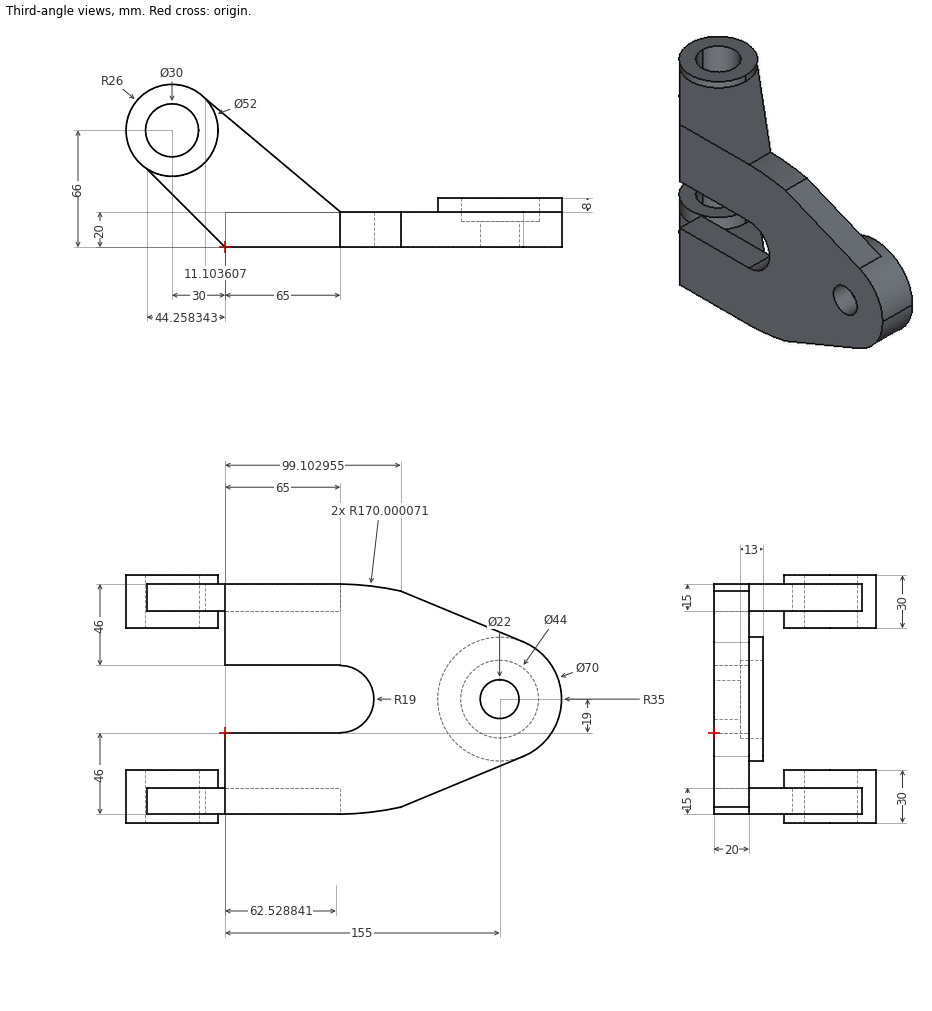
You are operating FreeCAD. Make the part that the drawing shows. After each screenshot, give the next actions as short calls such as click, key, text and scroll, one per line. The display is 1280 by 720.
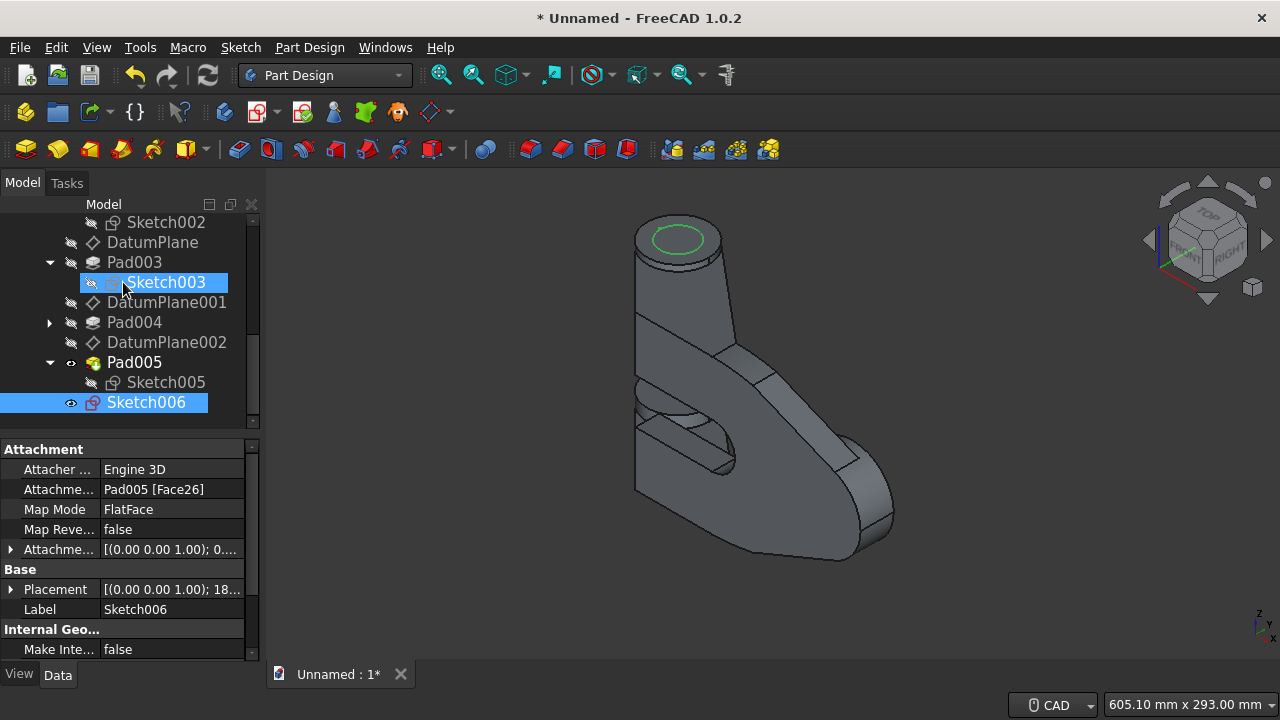
click(240, 150)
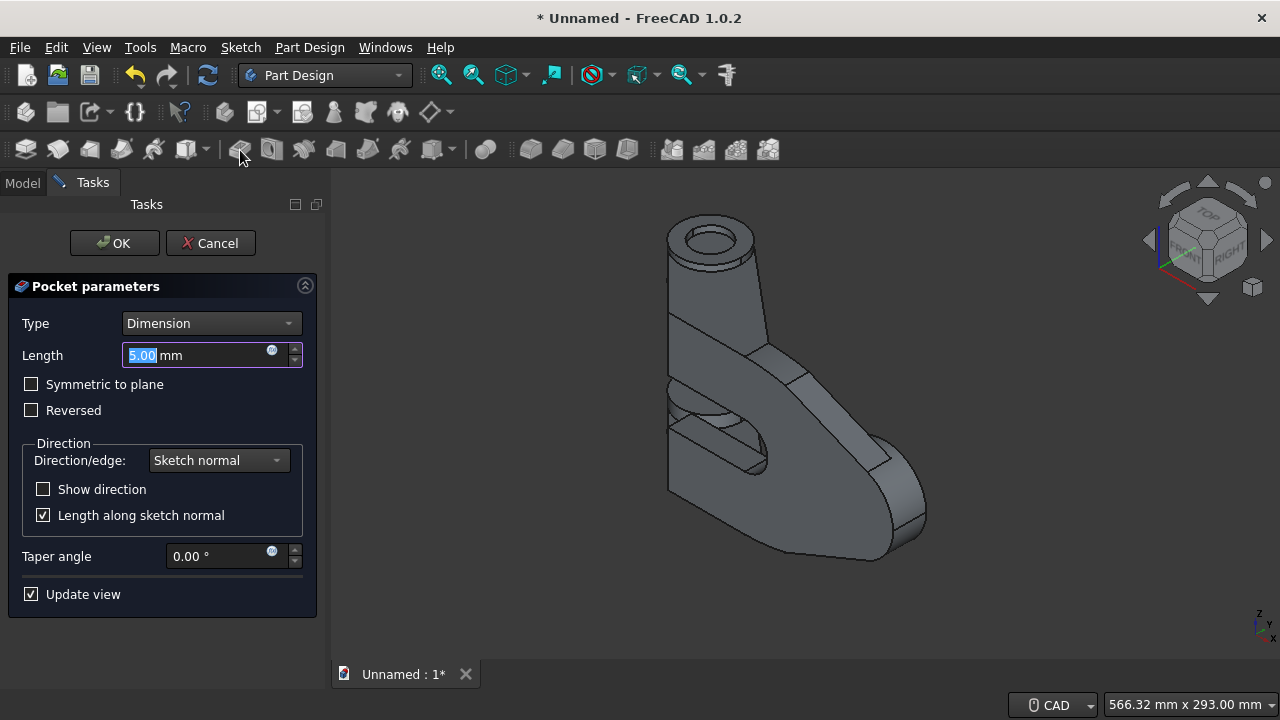
click(212, 324)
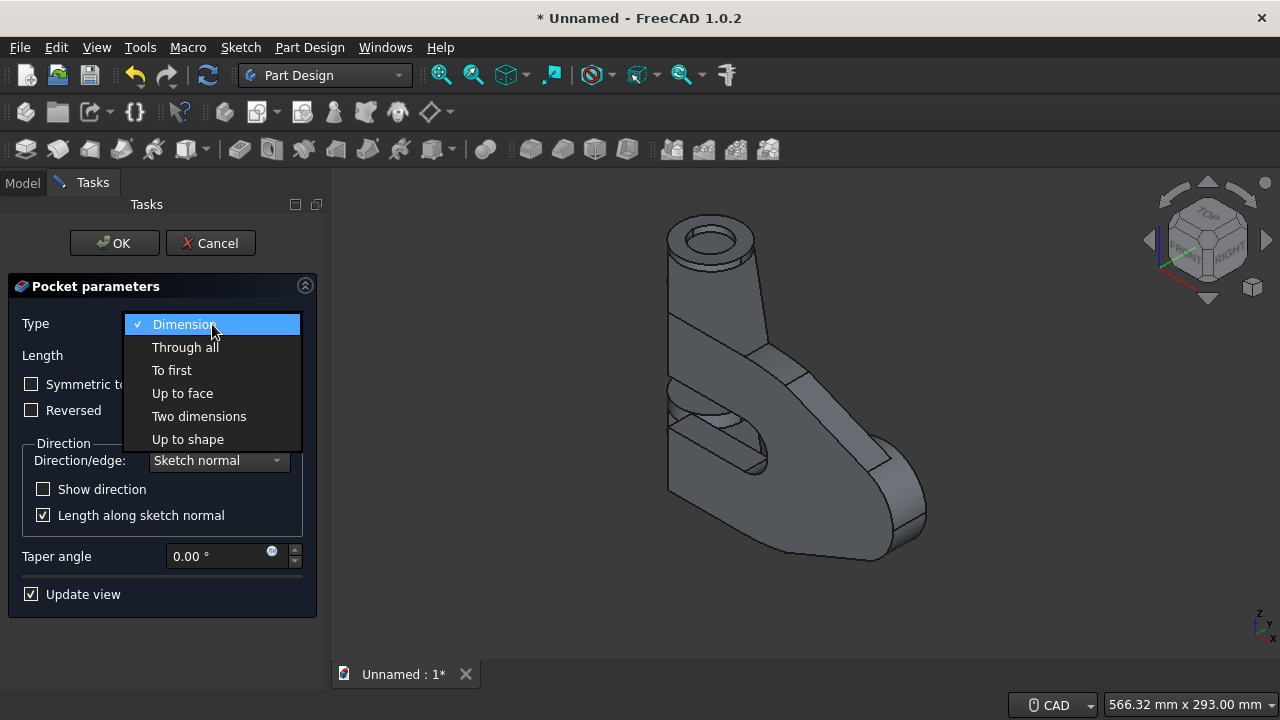
click(212, 348)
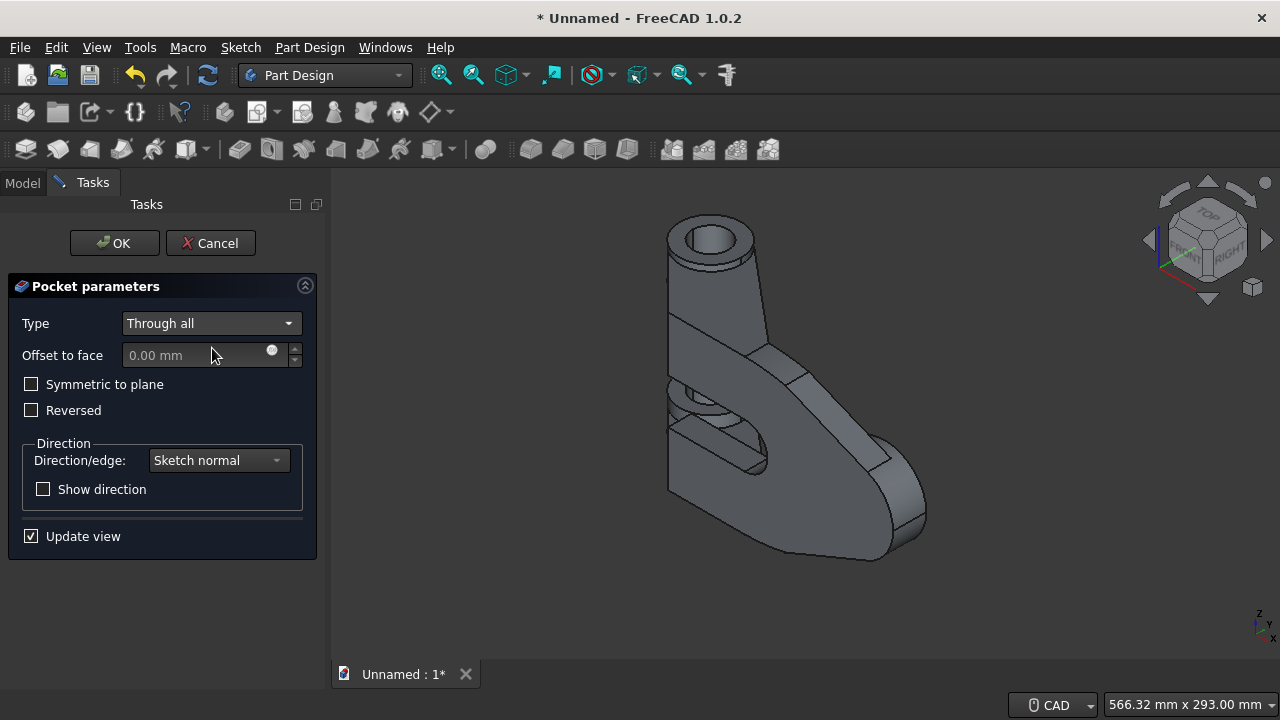
click(115, 243)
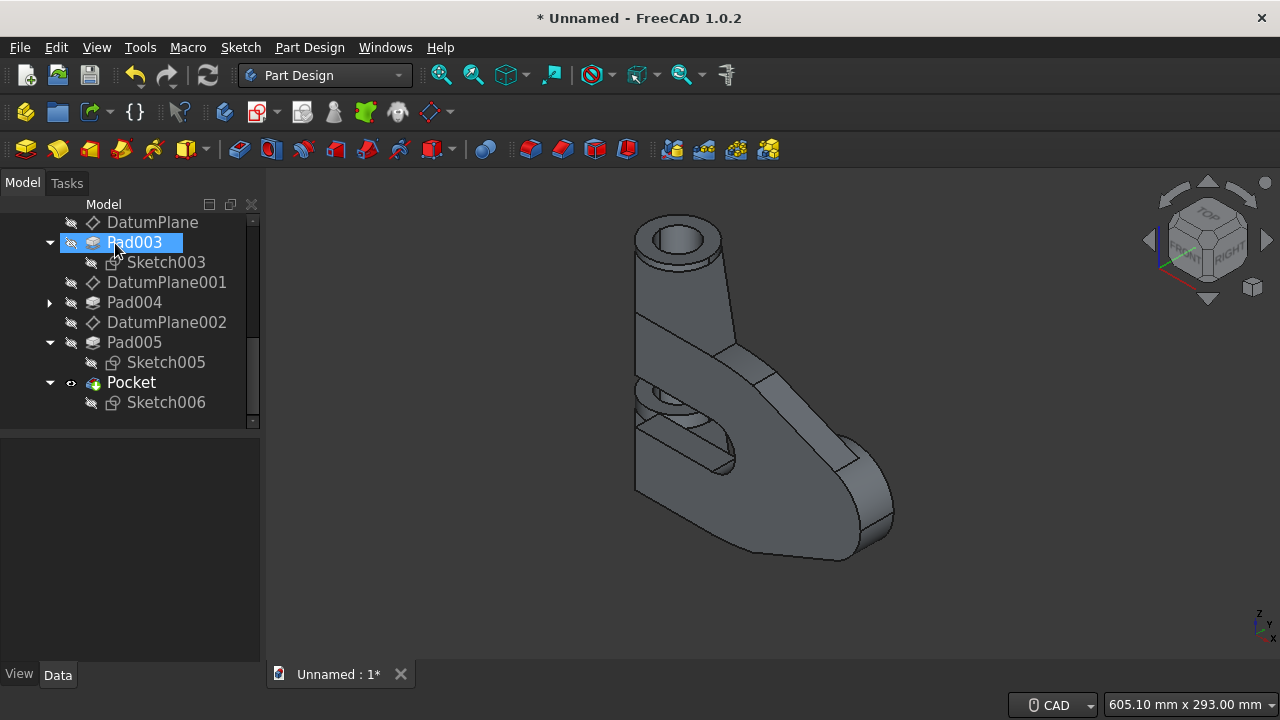
key(4)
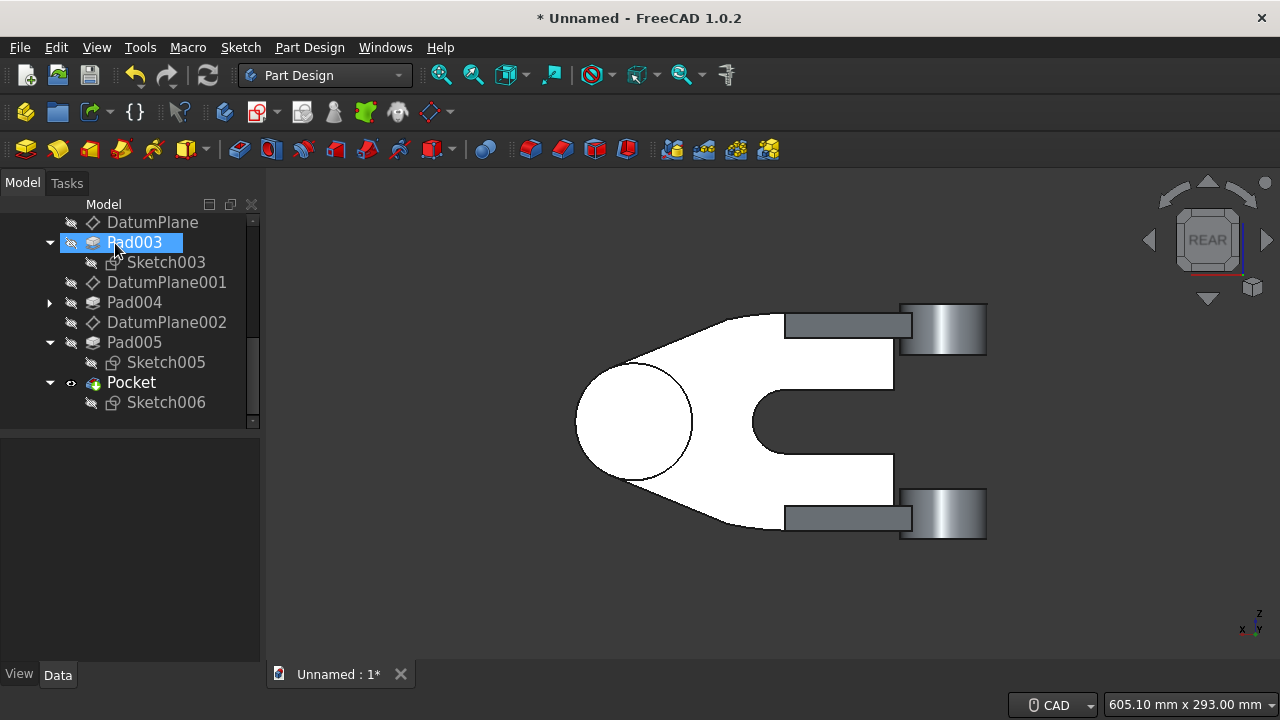
click(634, 421)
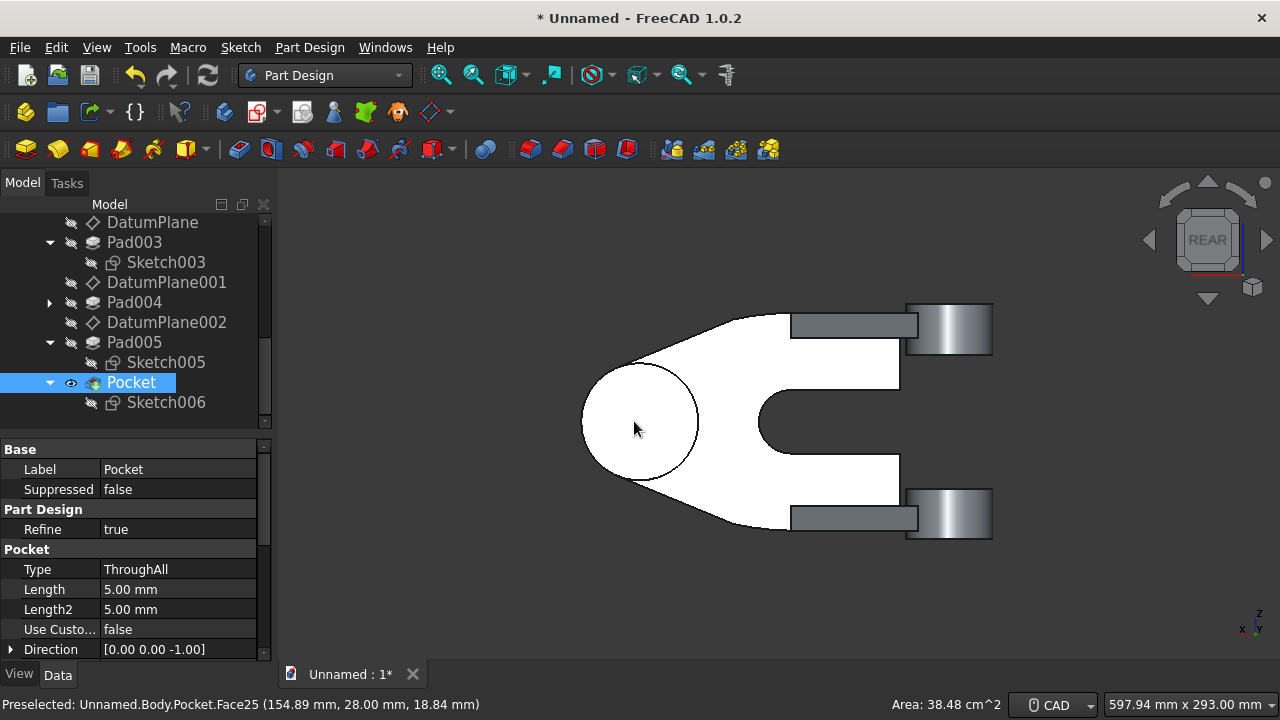
click(258, 112)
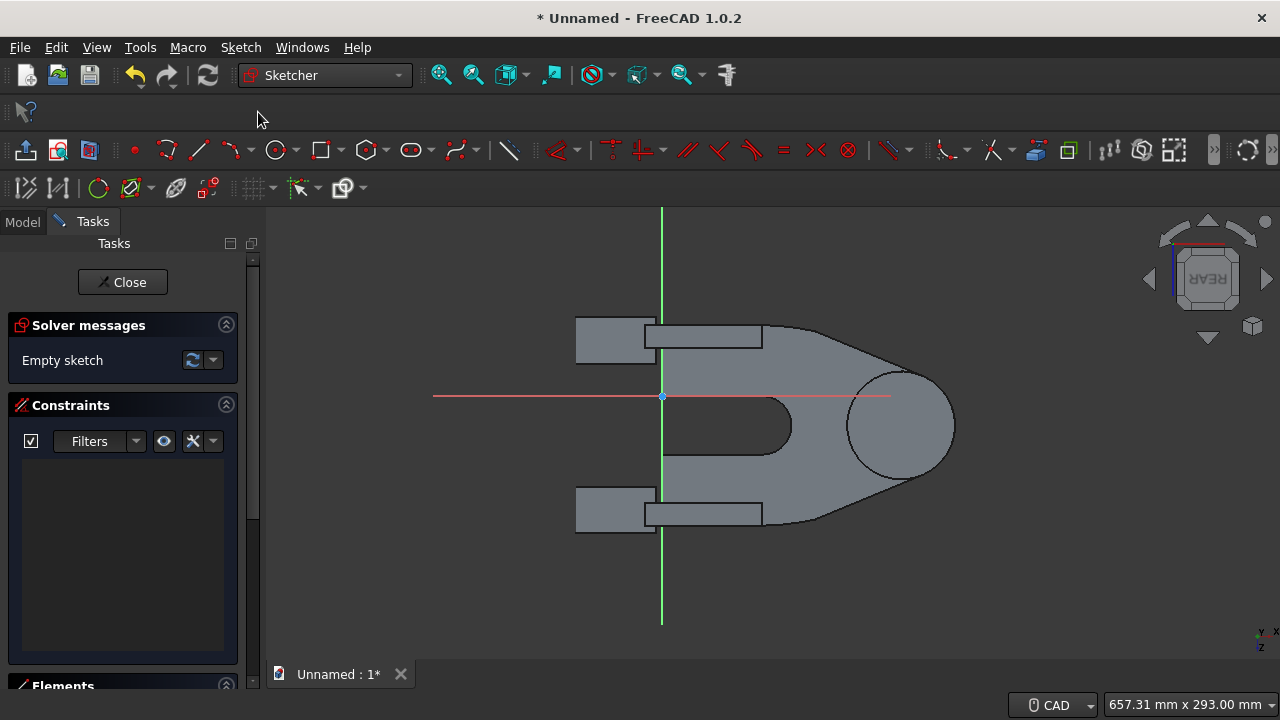
key(q)
key(s)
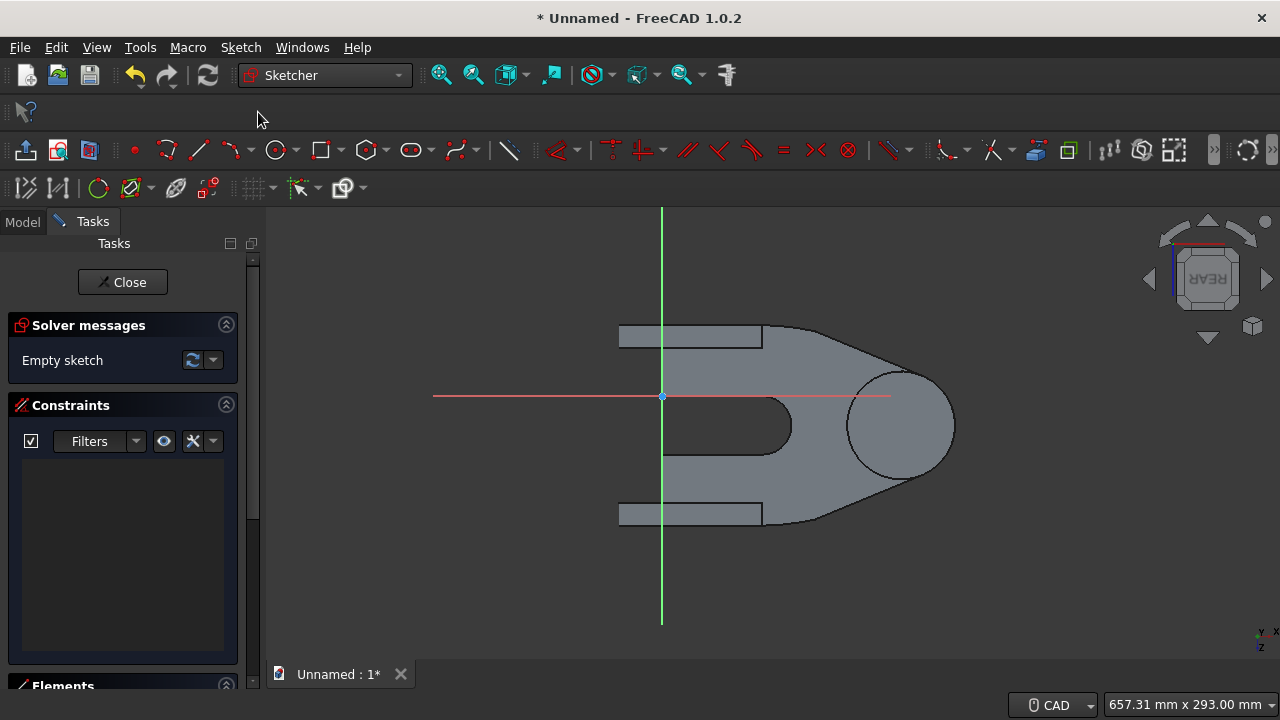
scroll(965, 423, up, 7)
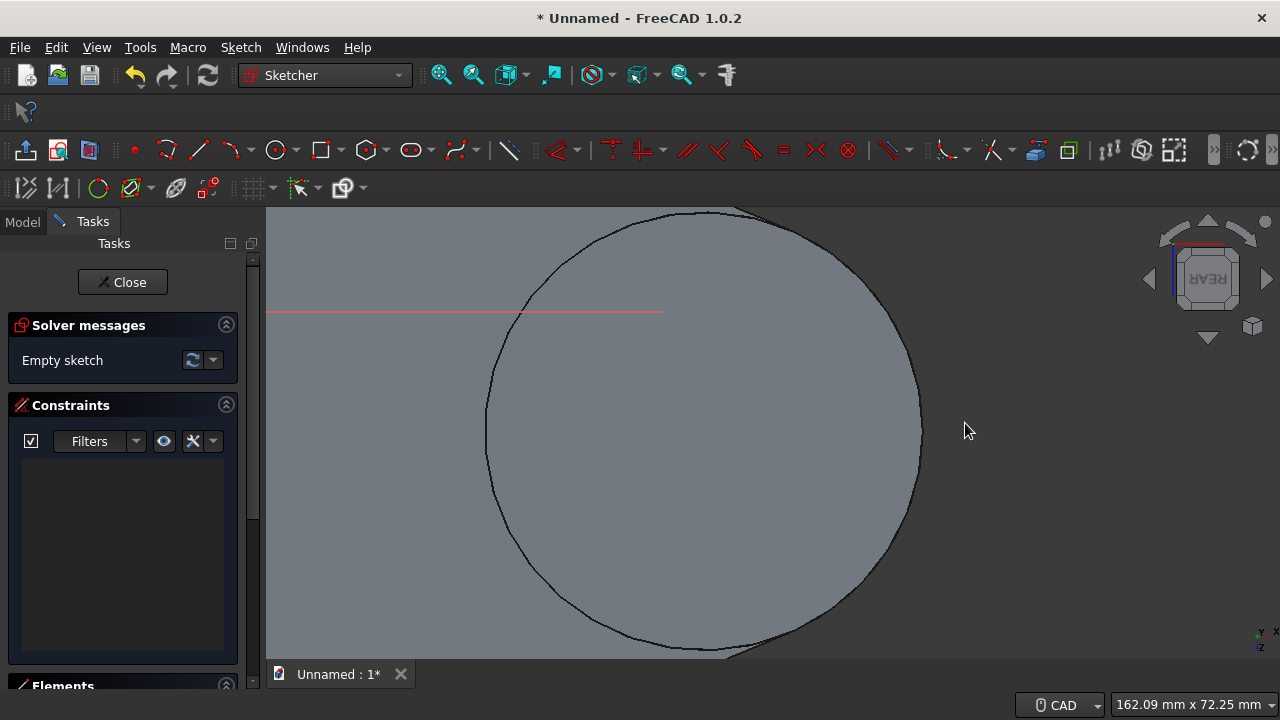
key(g)
key(c)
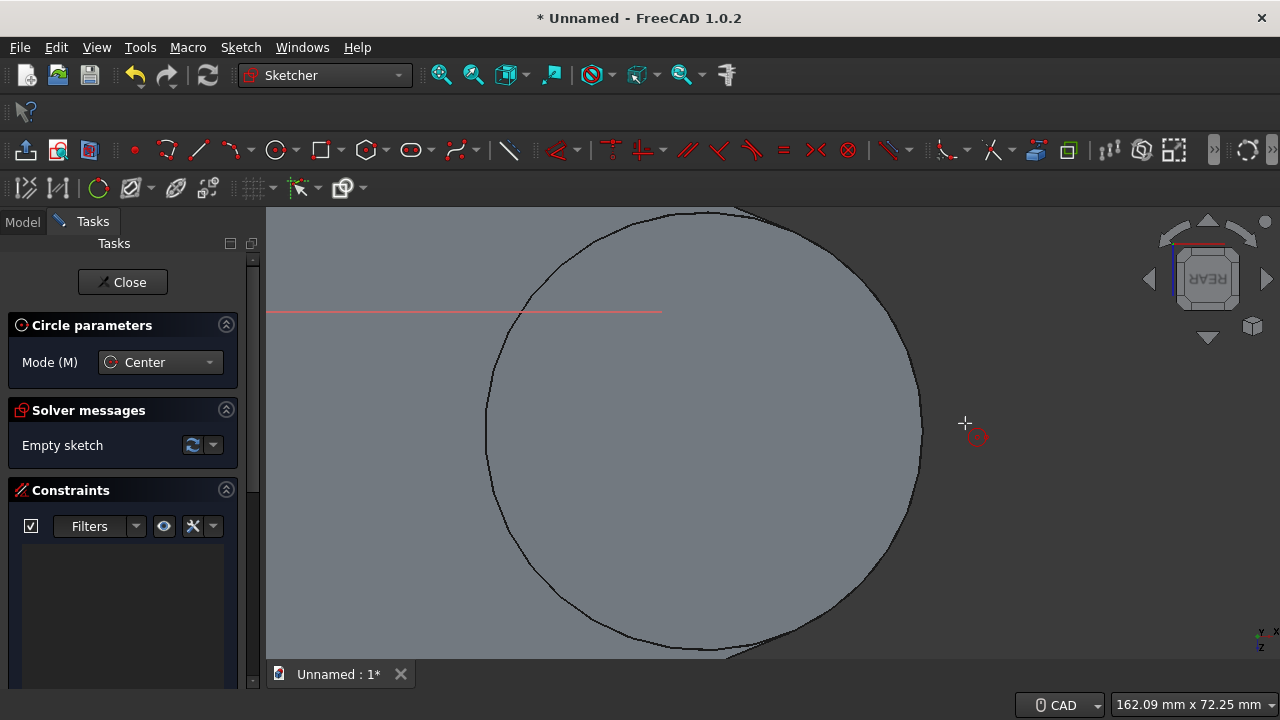
click(704, 431)
move(801, 334)